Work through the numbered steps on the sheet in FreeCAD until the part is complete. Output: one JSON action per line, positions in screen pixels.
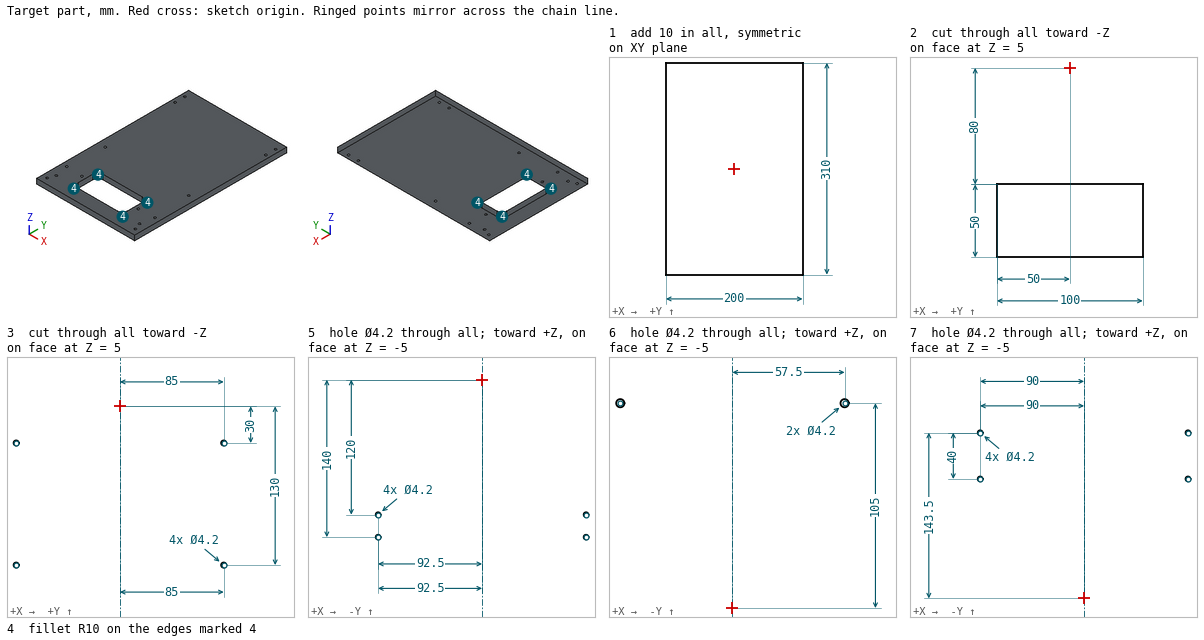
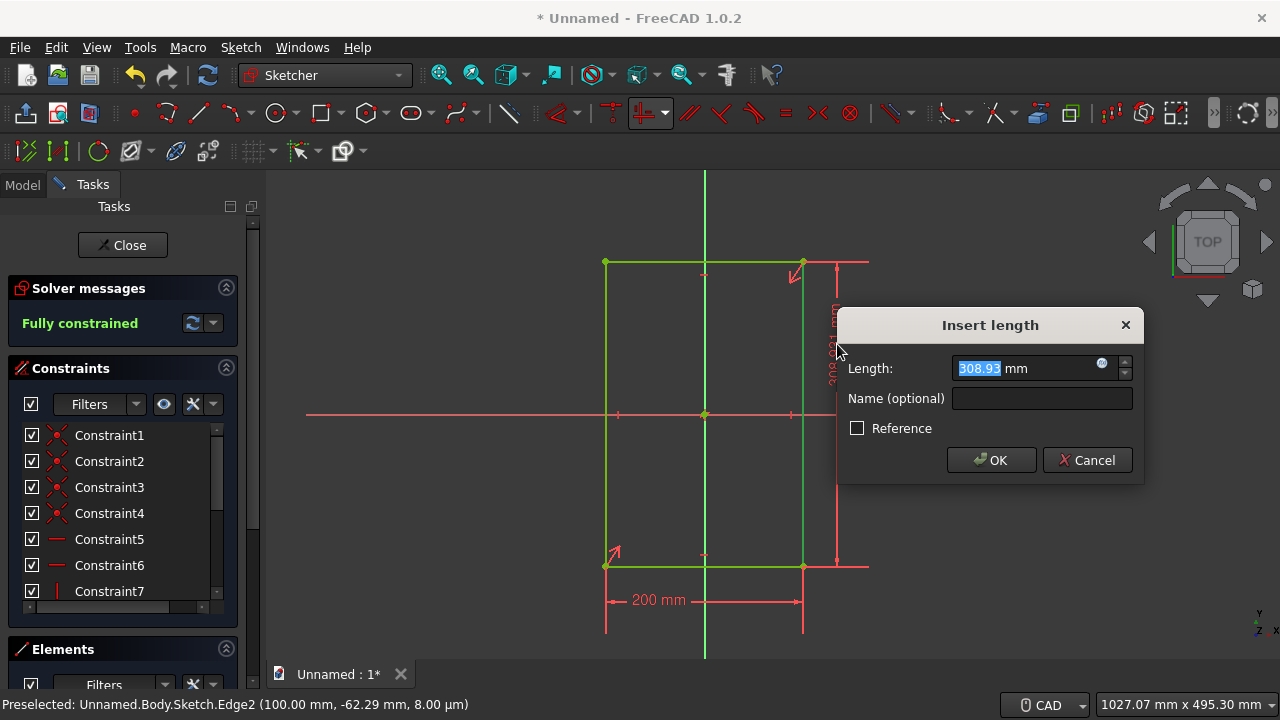
{"action": "type", "text": "310"}
{"action": "key", "text": "Return"}
{"action": "key", "text": "Escape"}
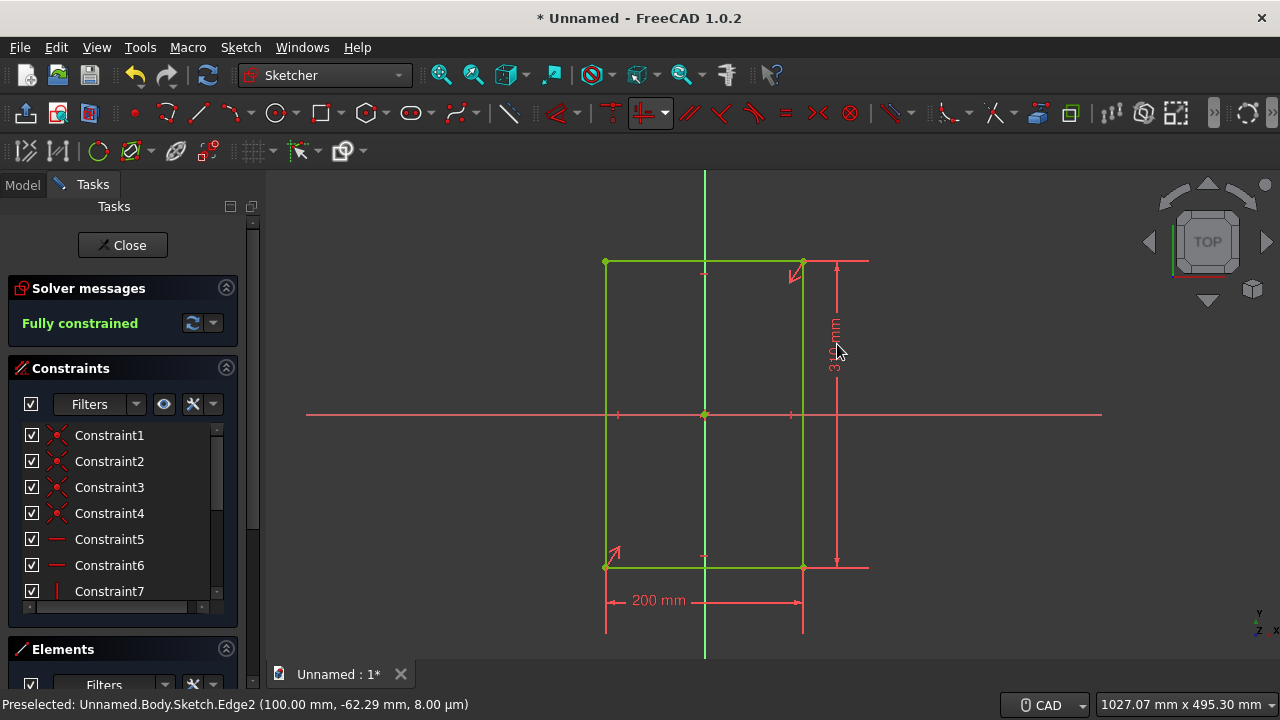
{"action": "left_click", "coordinate": [123, 245]}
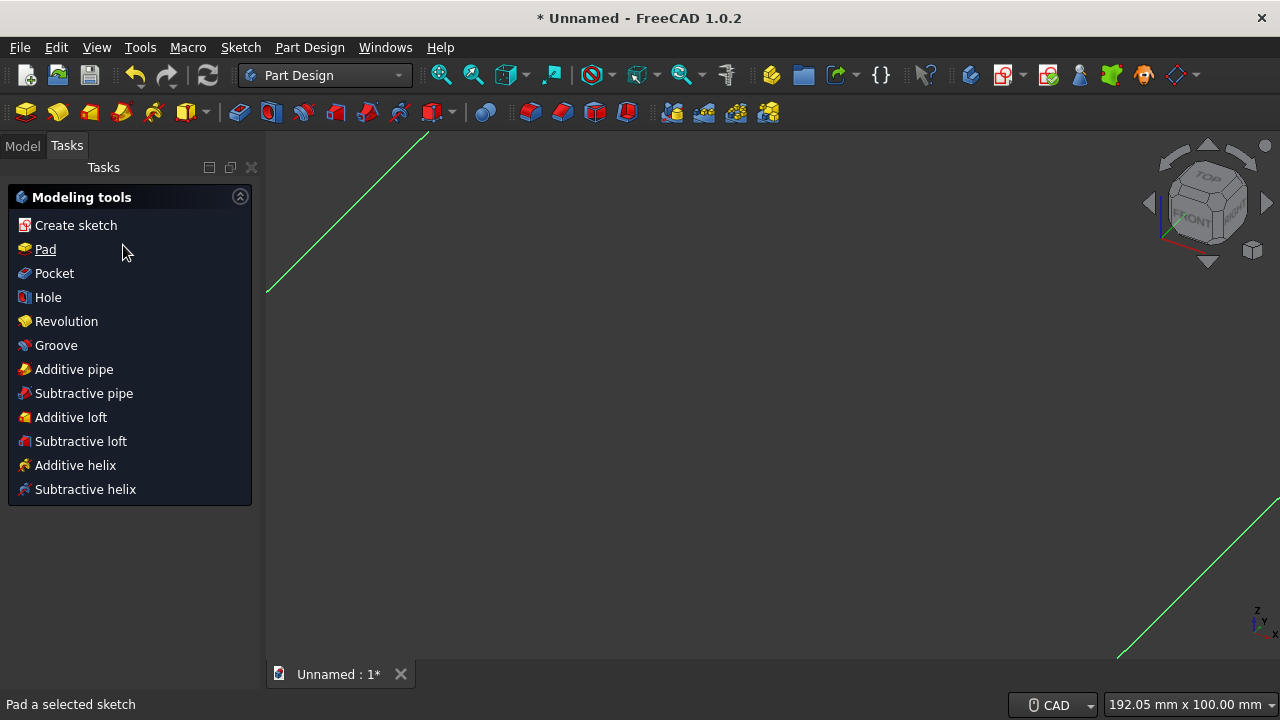
{"action": "left_click", "coordinate": [26, 112]}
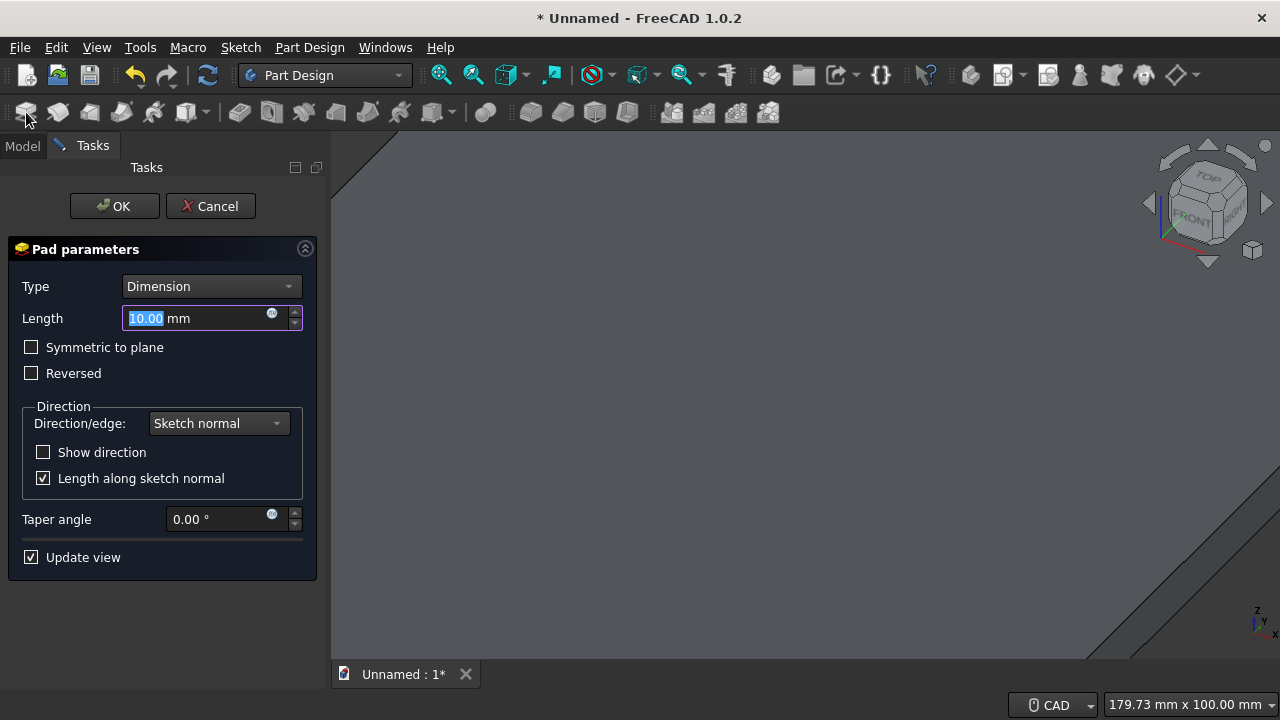
{"action": "type", "text": "10"}
{"action": "key", "text": "Tab"}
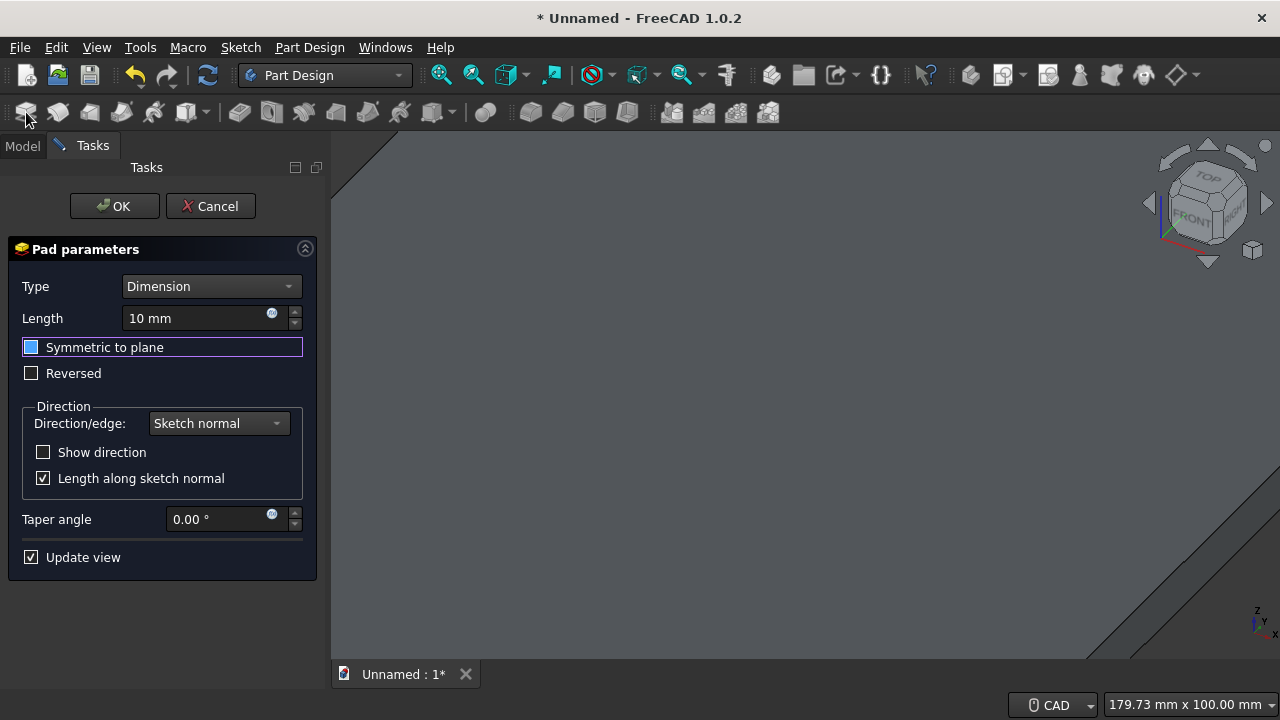
{"action": "left_click", "coordinate": [30, 347]}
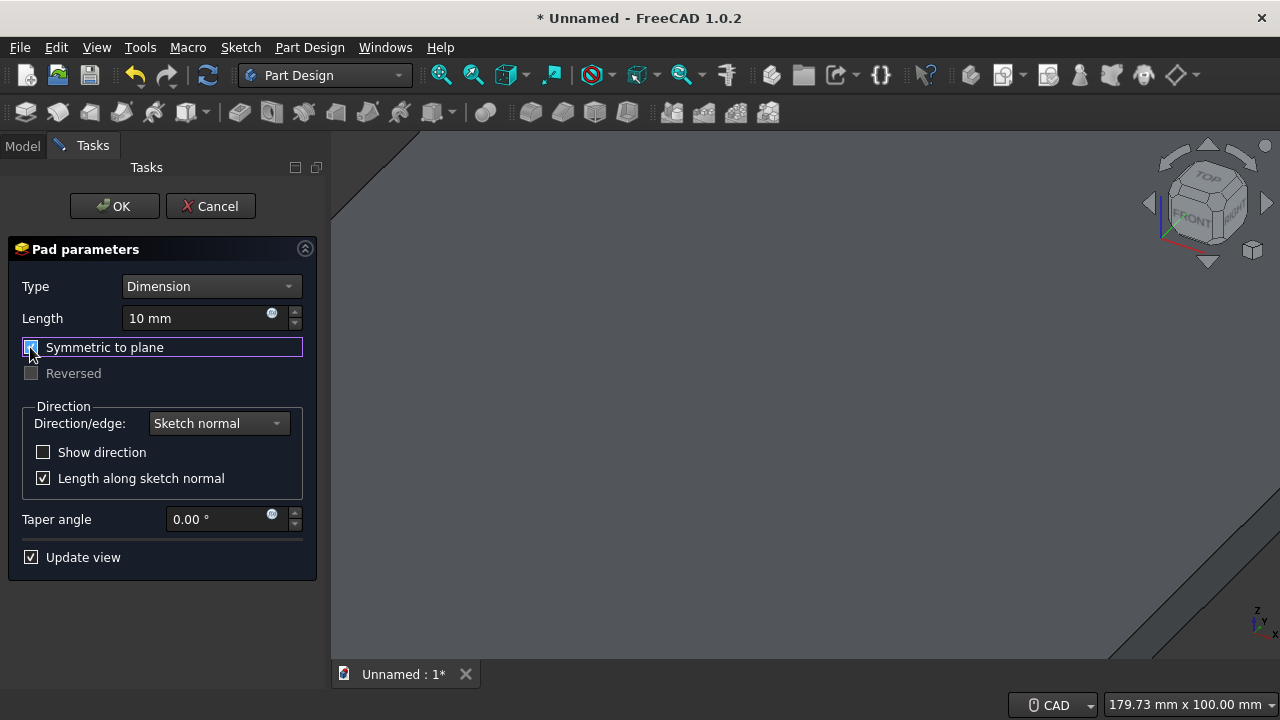
{"action": "left_click", "coordinate": [115, 206]}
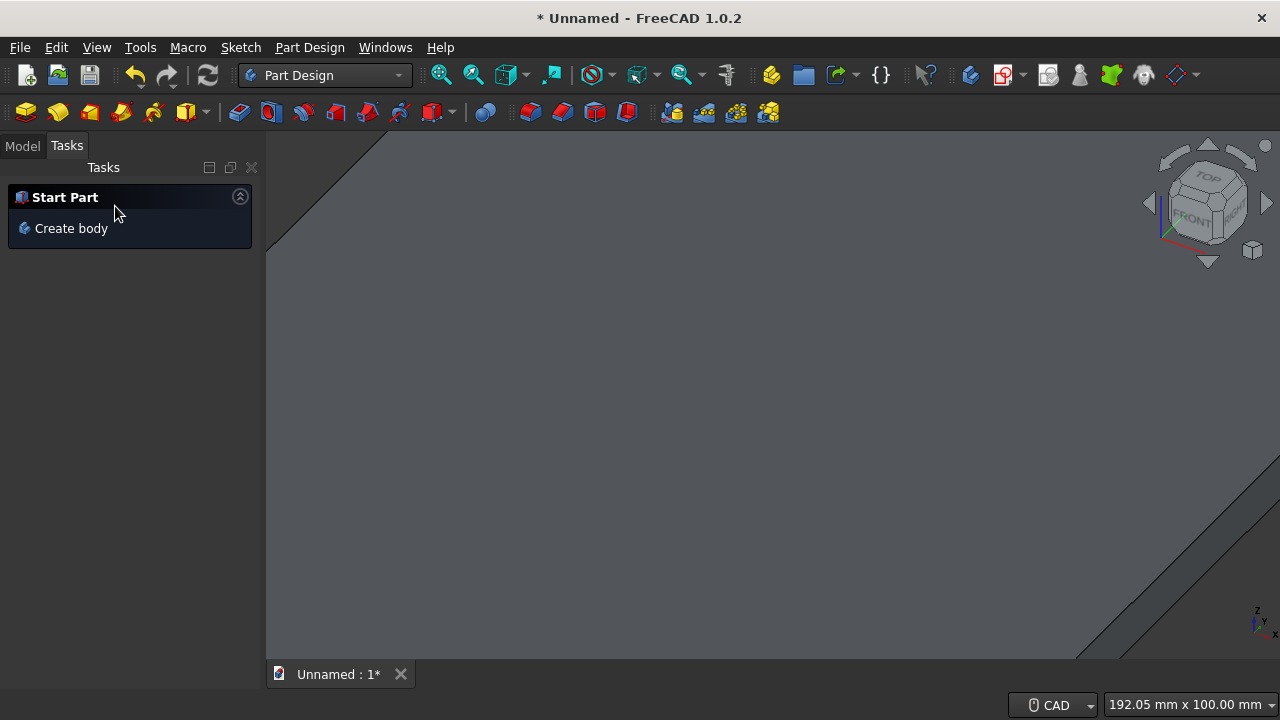
{"action": "left_click", "coordinate": [442, 76]}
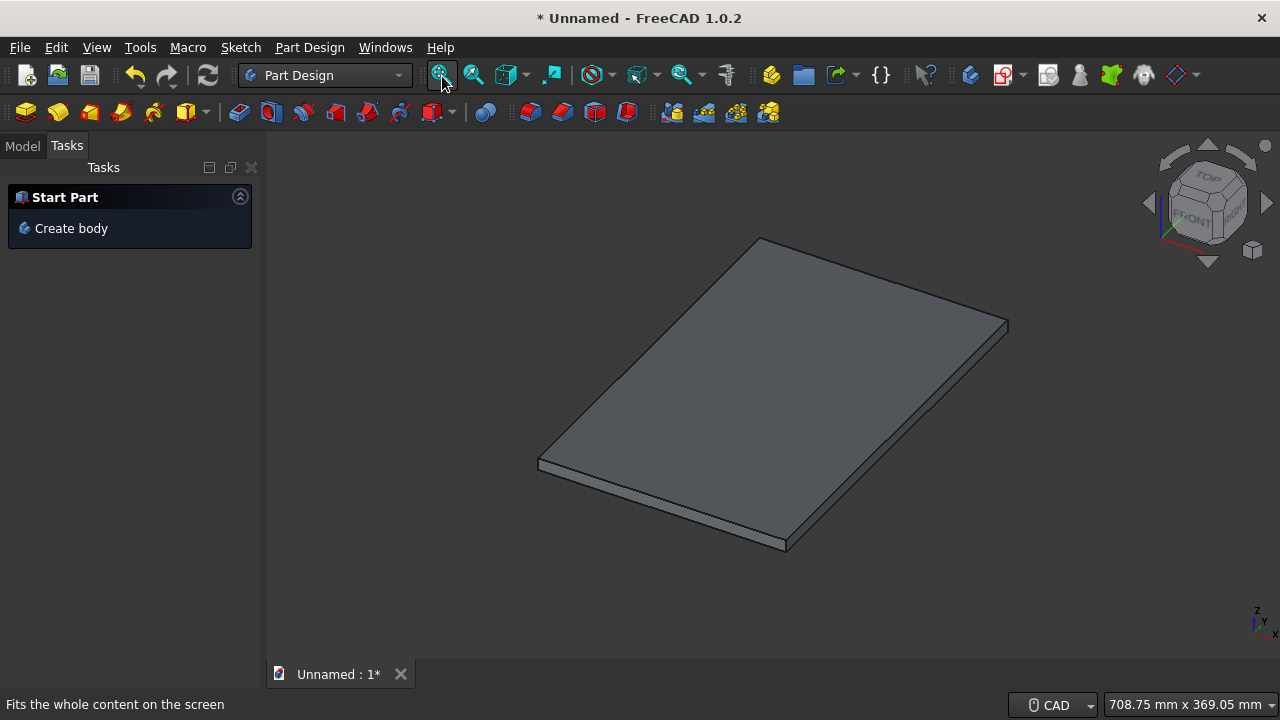
{"action": "left_click", "coordinate": [805, 357]}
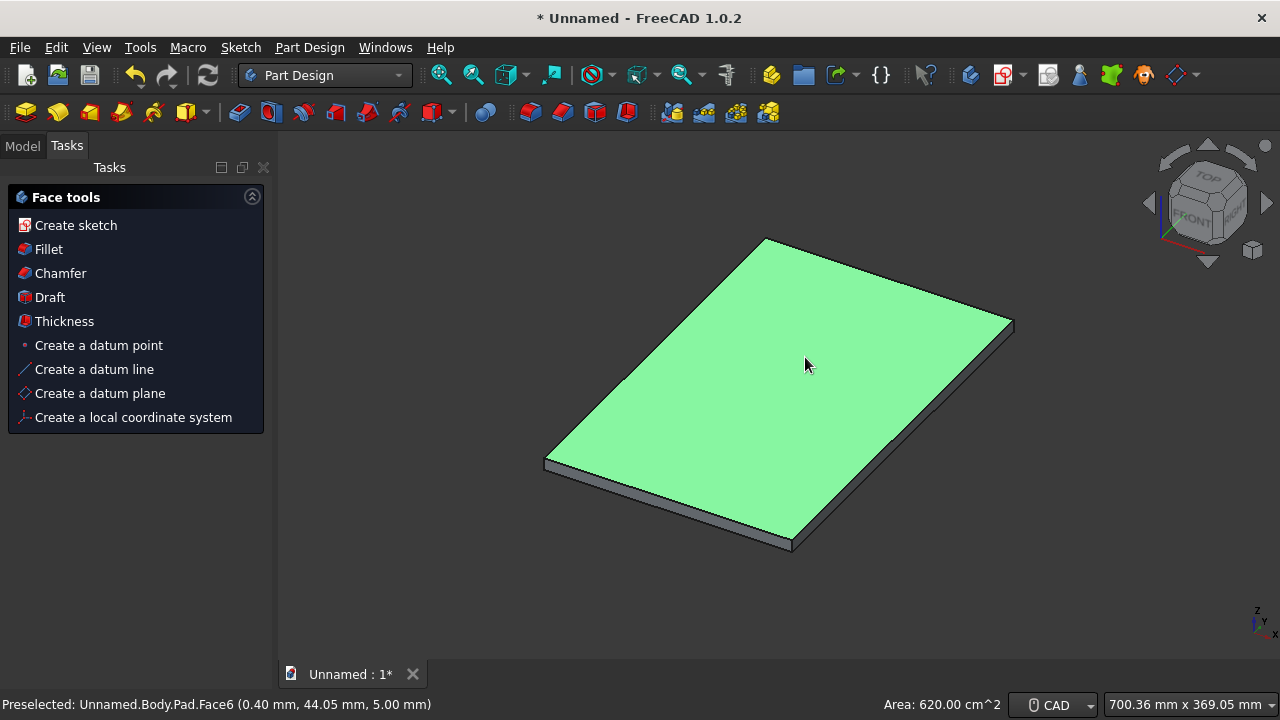
{"action": "left_click", "coordinate": [1004, 76]}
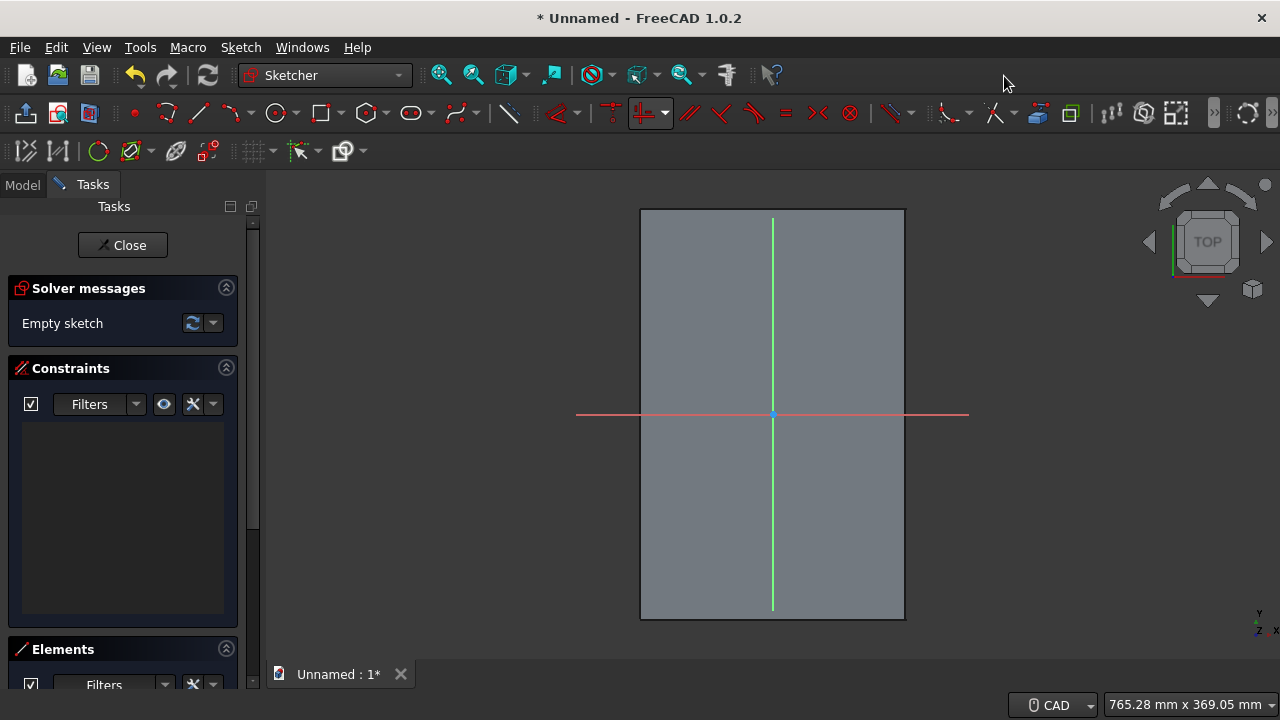
{"action": "scroll", "coordinate": [856, 605], "scroll_direction": "up", "scroll_amount": 3}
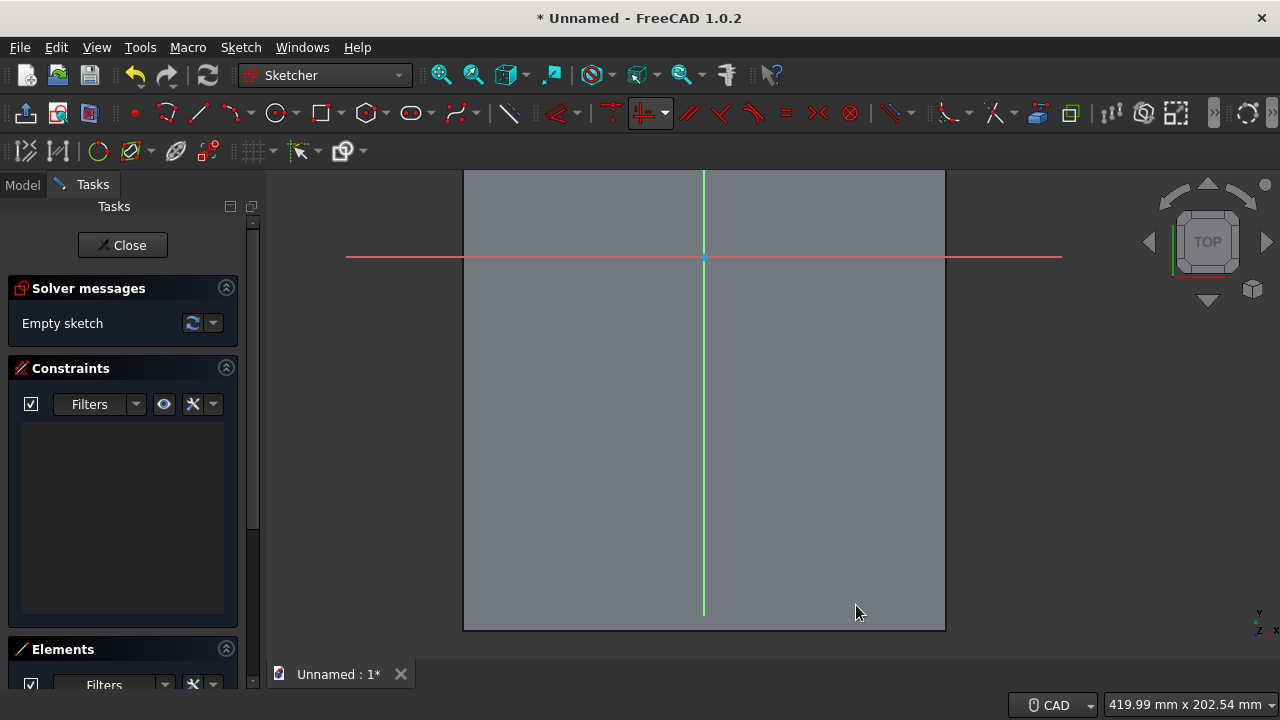
{"action": "left_click", "coordinate": [322, 114]}